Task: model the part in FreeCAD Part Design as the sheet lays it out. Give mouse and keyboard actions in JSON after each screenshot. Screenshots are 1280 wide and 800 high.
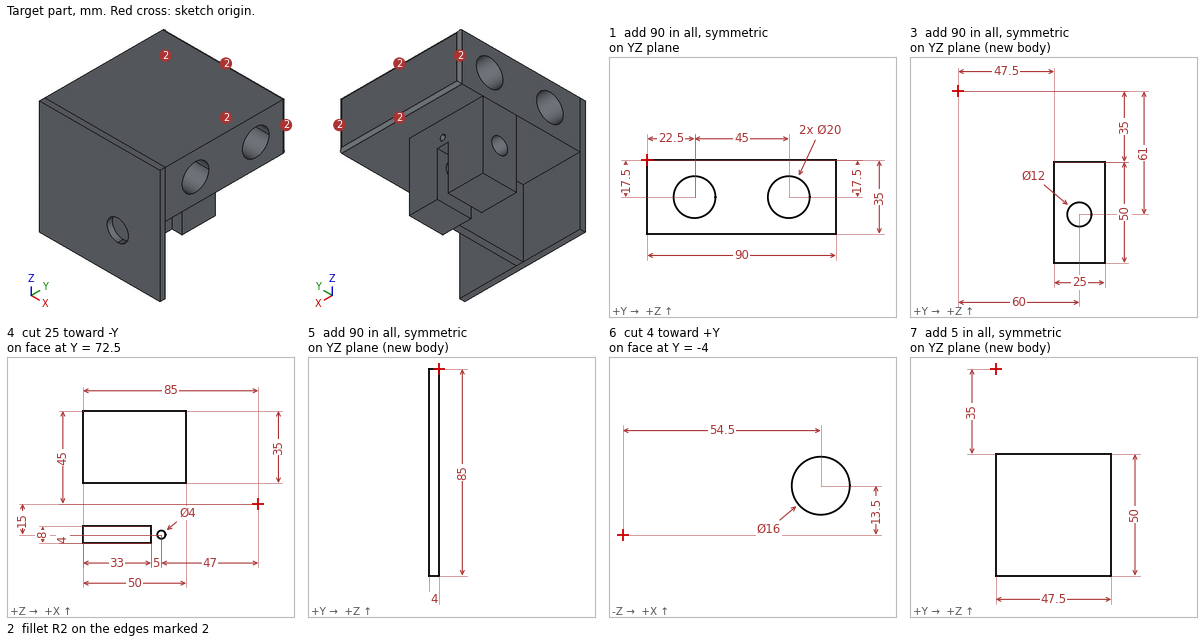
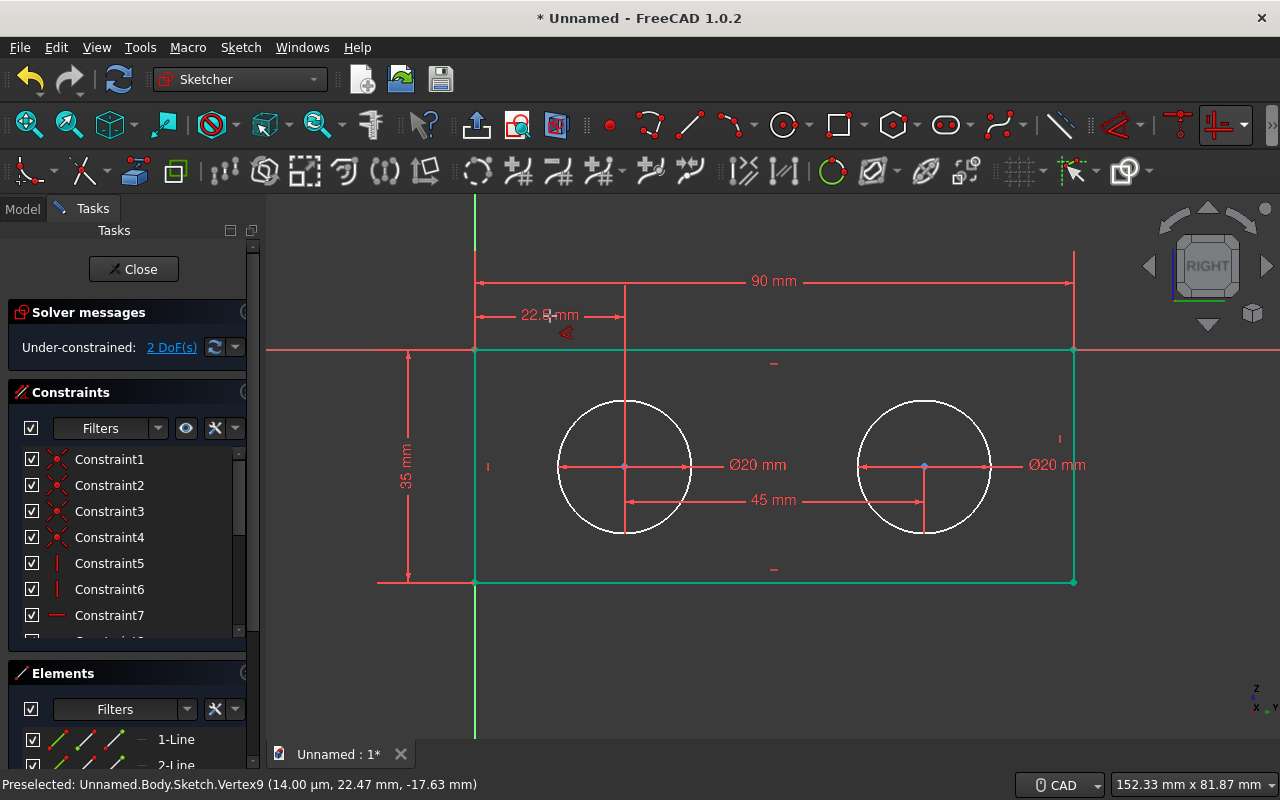
{"action": "left_click", "coordinate": [625, 467]}
{"action": "left_click", "coordinate": [441, 408]}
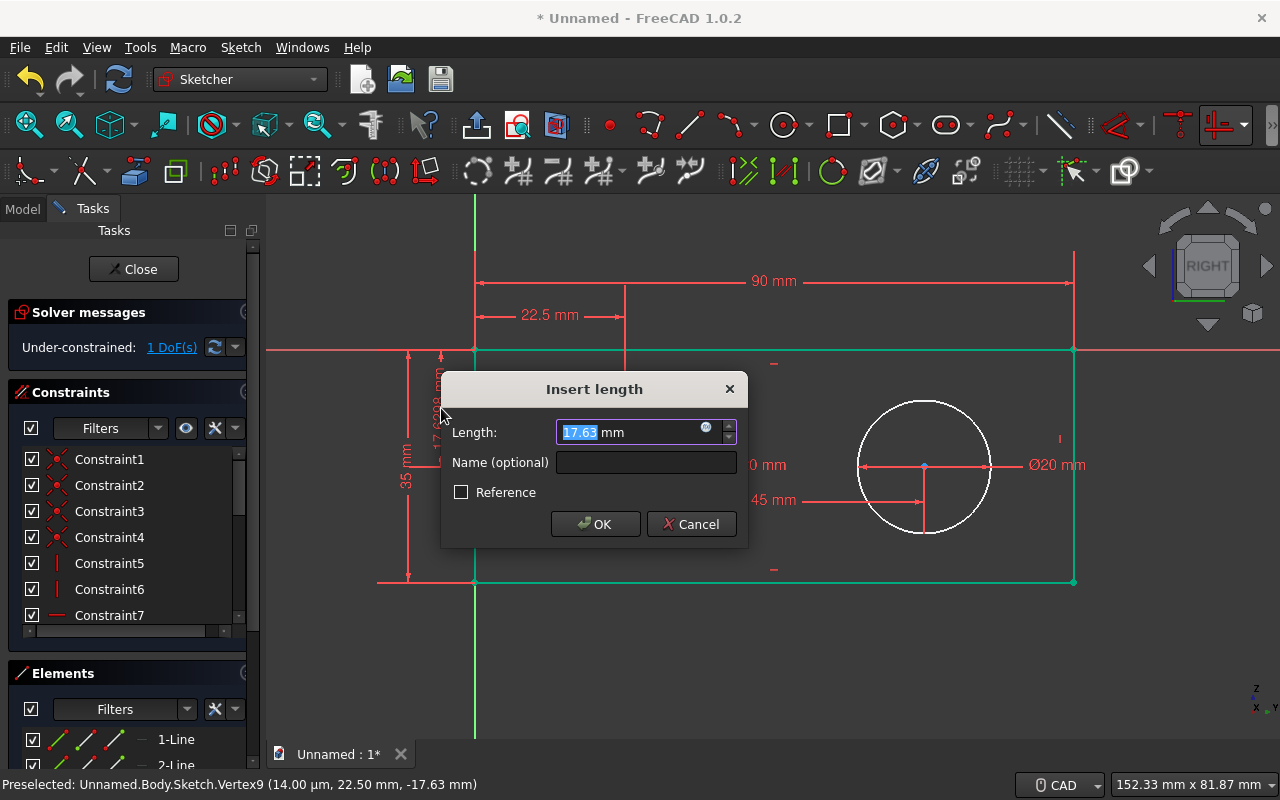
{"action": "type", "text": "17.5"}
{"action": "key", "text": "Return"}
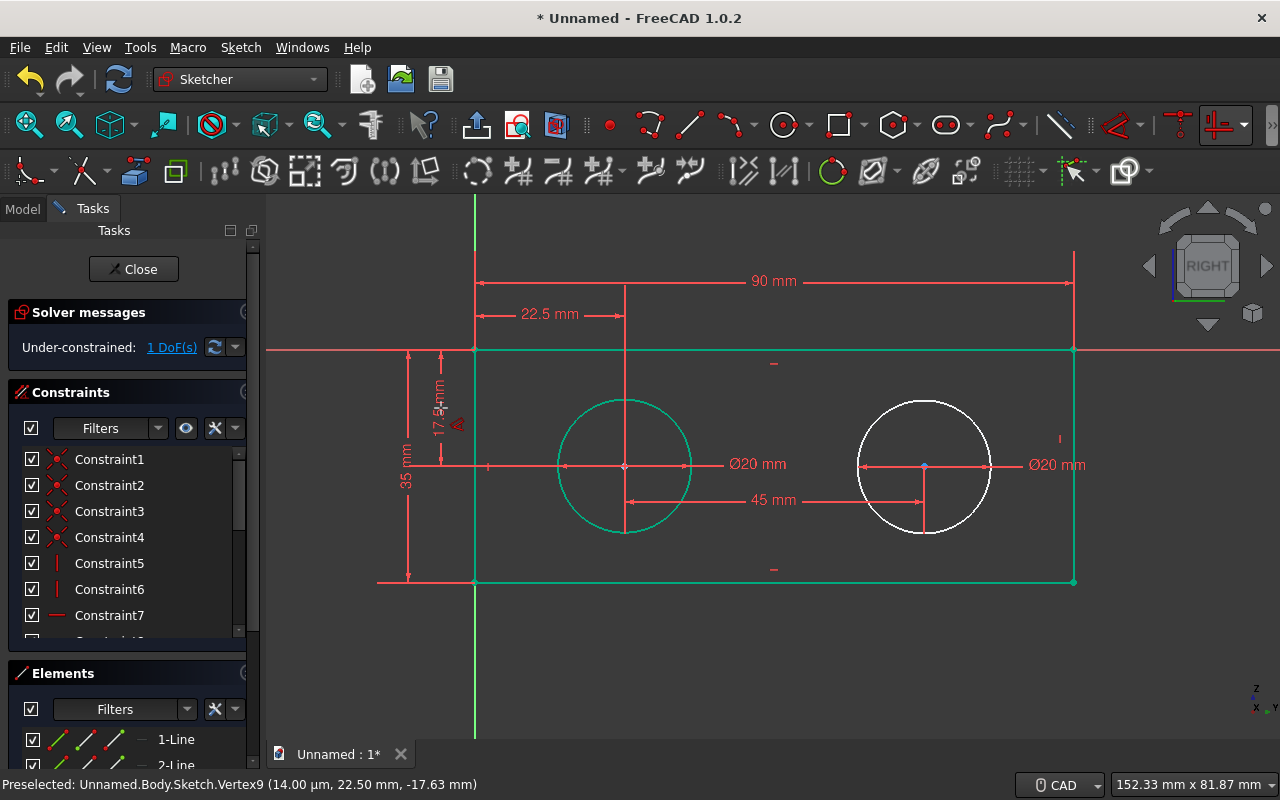
{"action": "left_click", "coordinate": [924, 467]}
{"action": "left_click", "coordinate": [441, 381]}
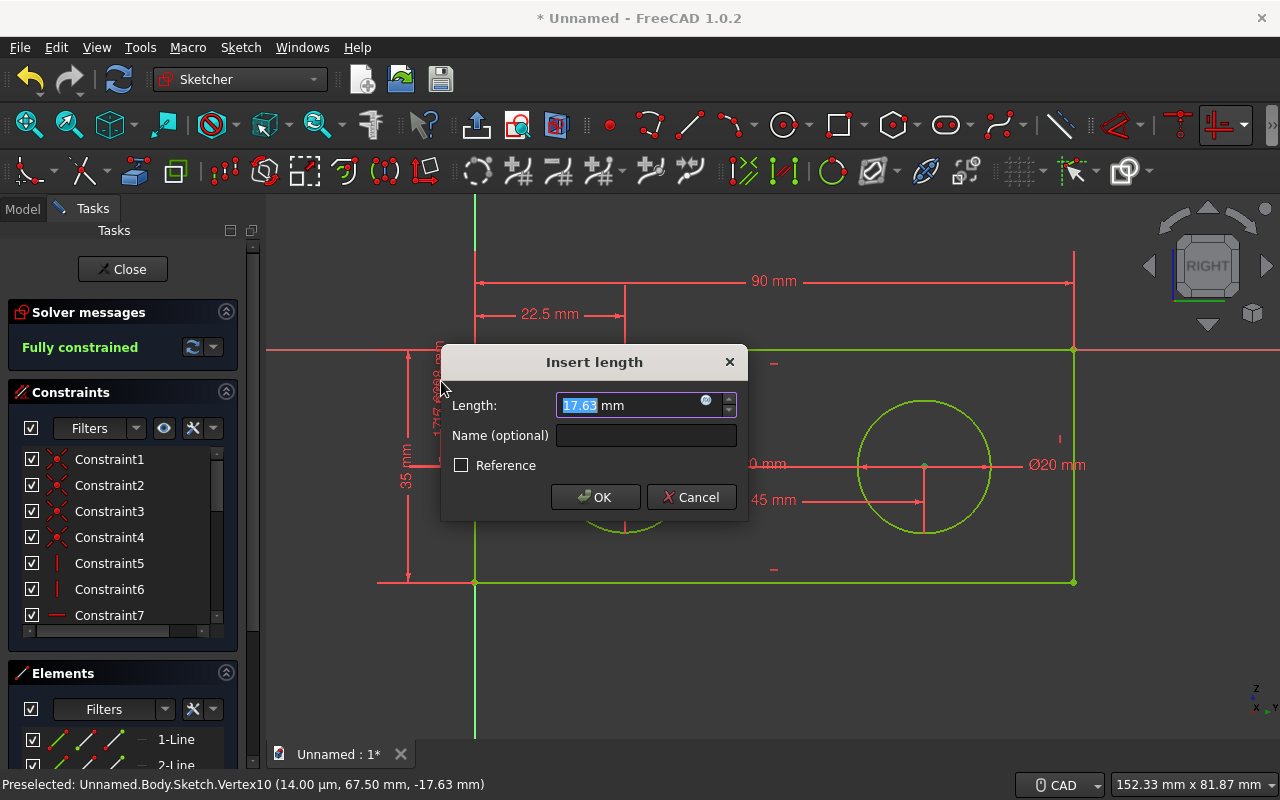
{"action": "type", "text": "17.5"}
{"action": "key", "text": "Return"}
{"action": "key", "text": "Escape"}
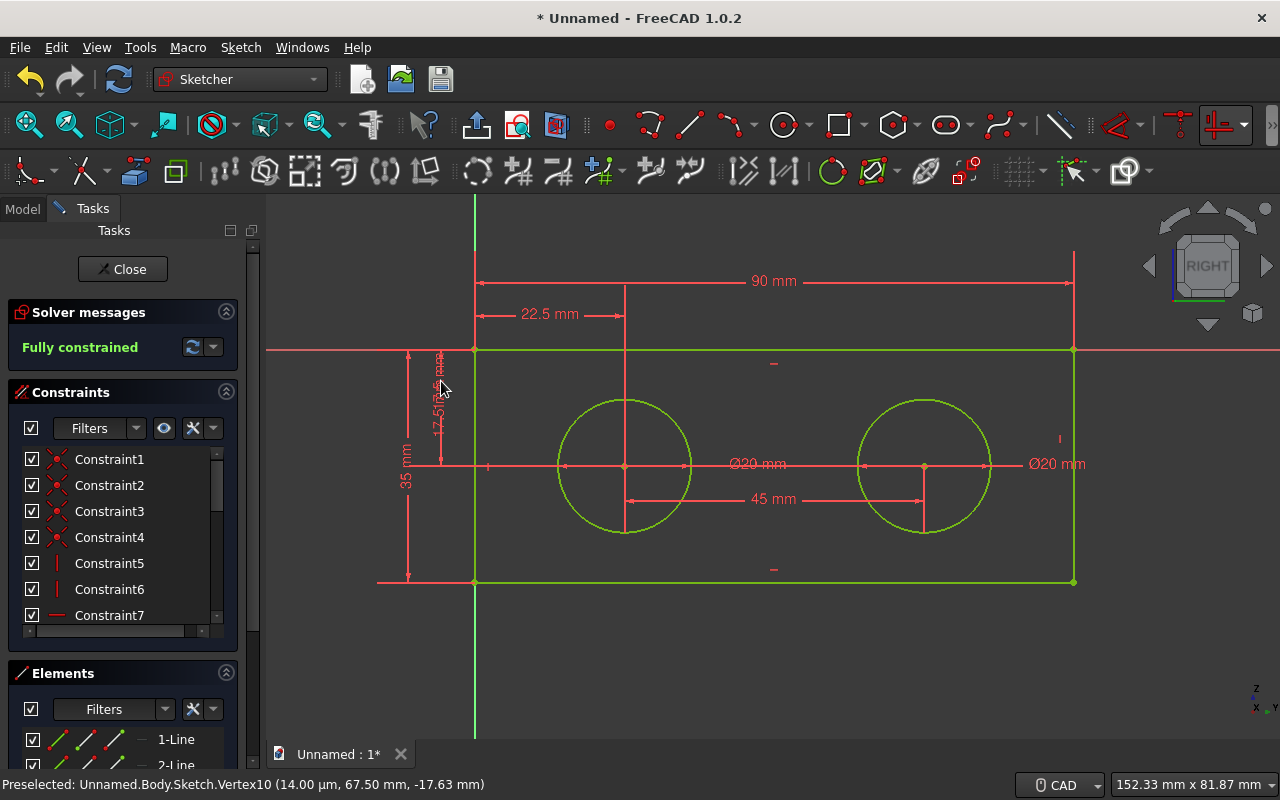
{"action": "left_click", "coordinate": [123, 269]}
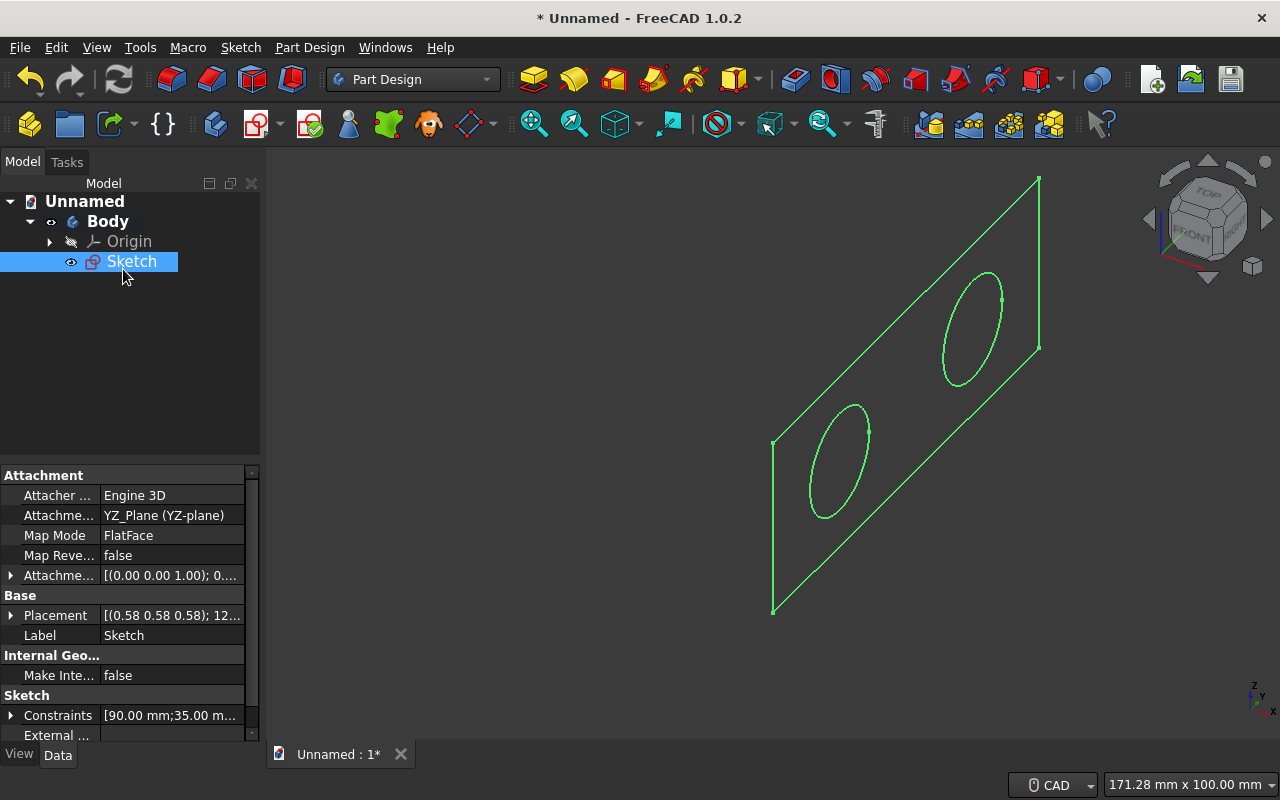
{"action": "left_click", "coordinate": [534, 80]}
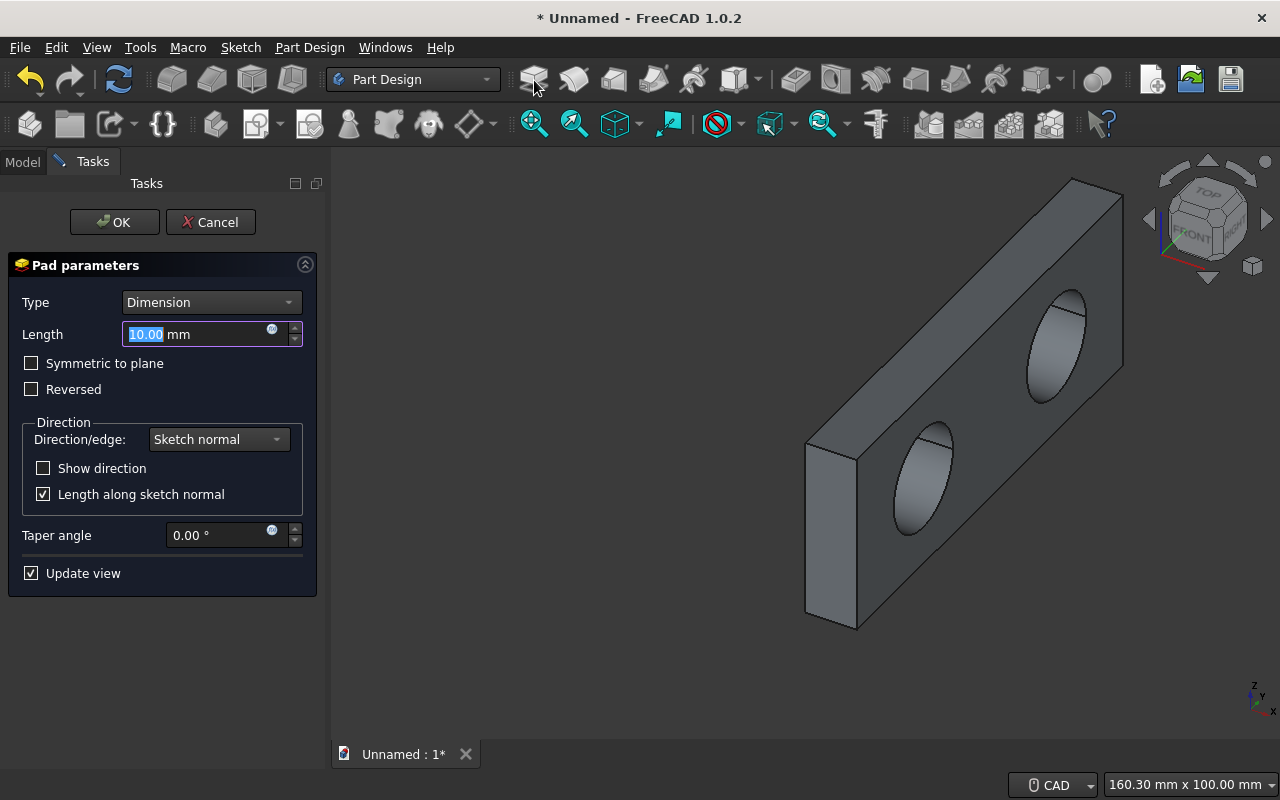
{"action": "type", "text": "90"}
{"action": "key", "text": "Tab"}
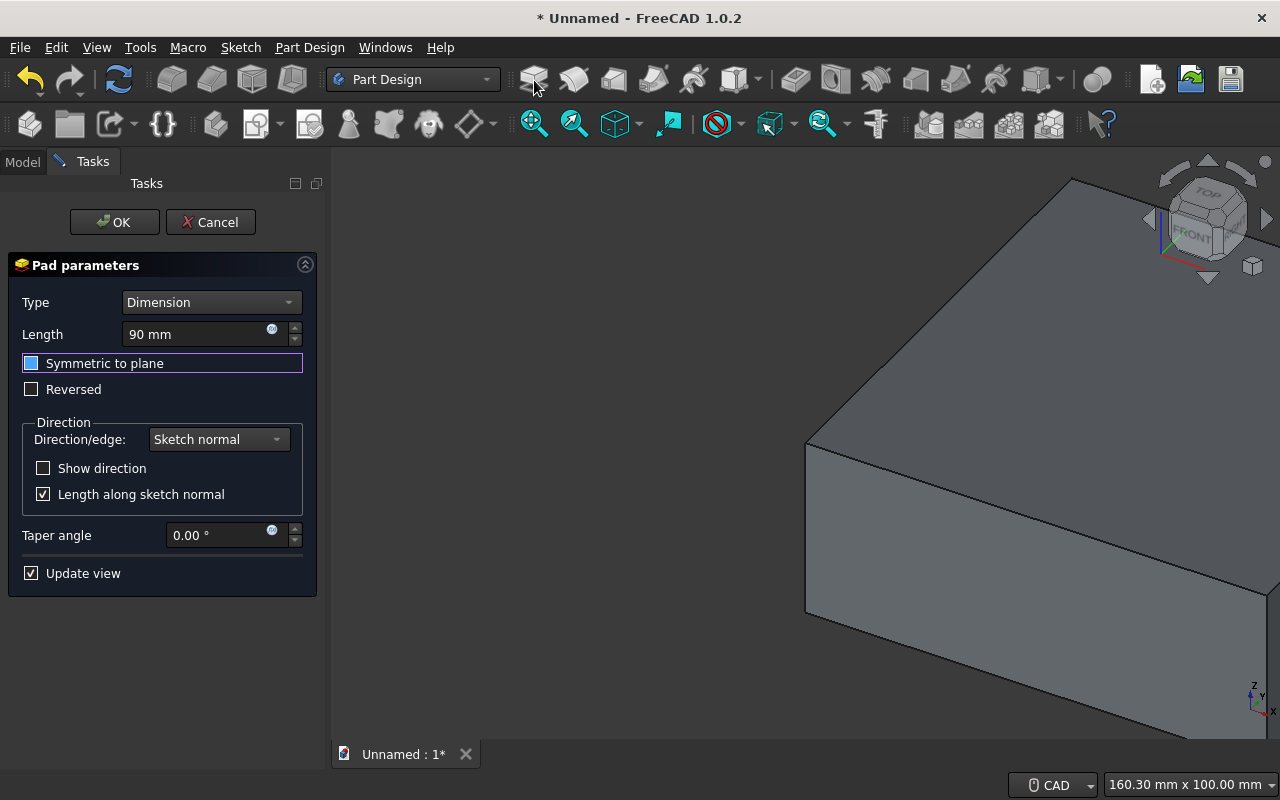
{"action": "left_click", "coordinate": [30, 363]}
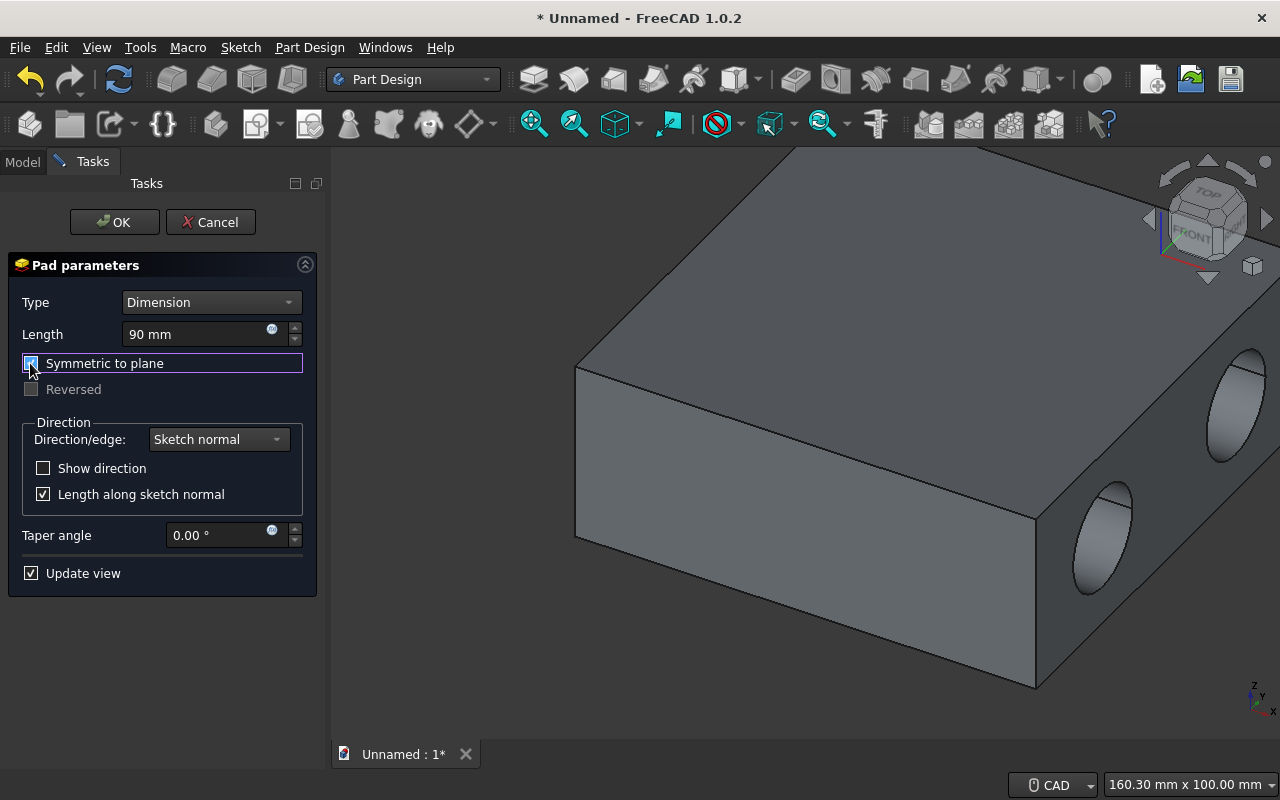
{"action": "left_click", "coordinate": [115, 222]}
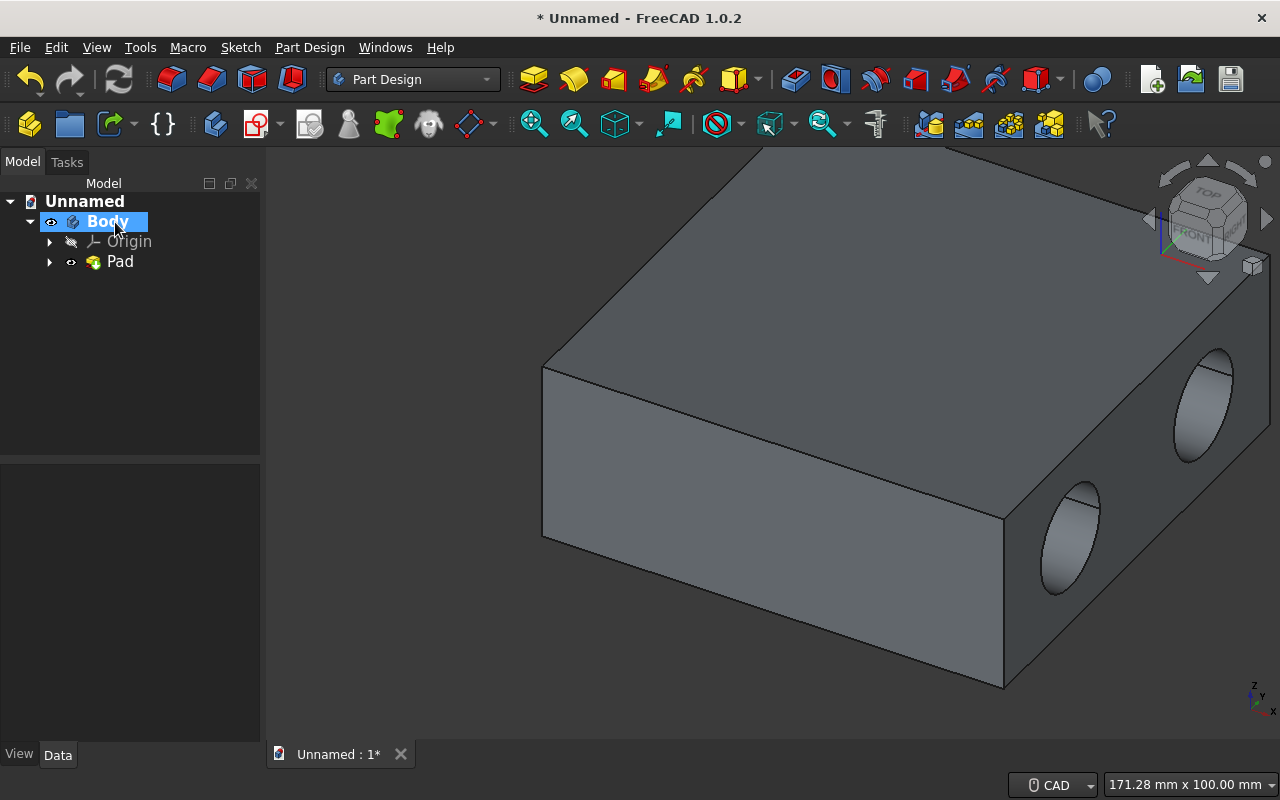
{"action": "left_click", "coordinate": [536, 124]}